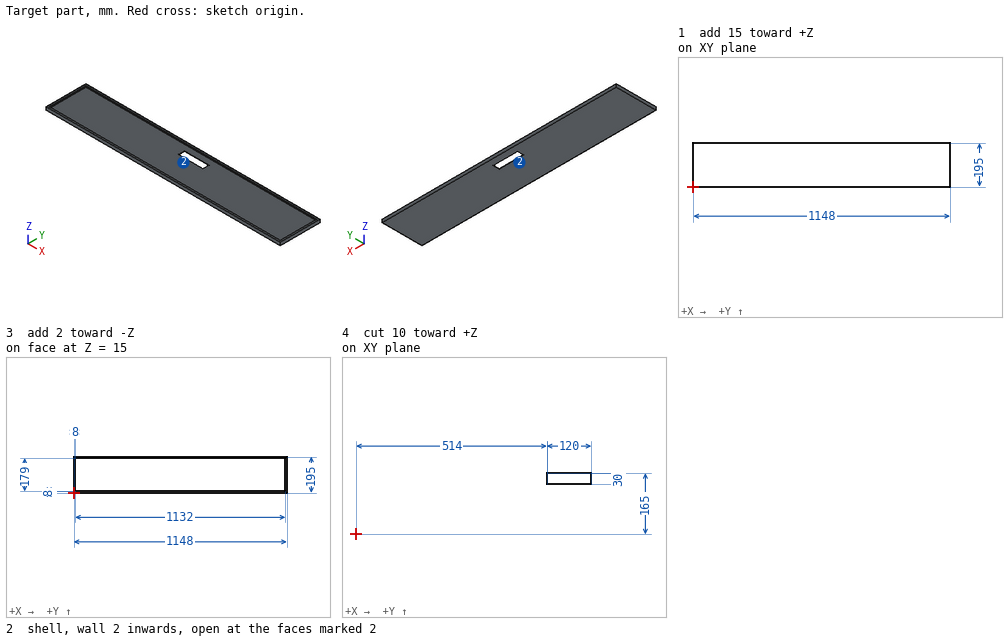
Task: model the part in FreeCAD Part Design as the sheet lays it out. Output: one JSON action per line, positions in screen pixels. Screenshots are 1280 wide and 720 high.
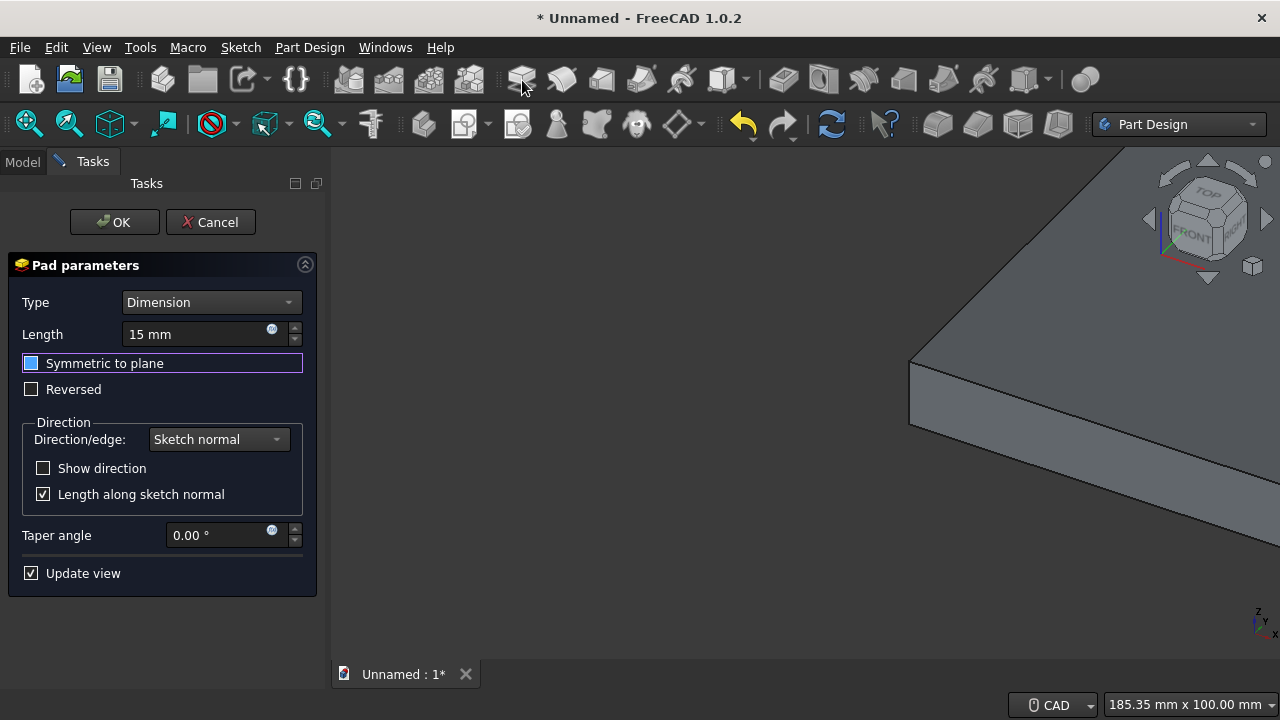
{"action": "left_click", "coordinate": [115, 222]}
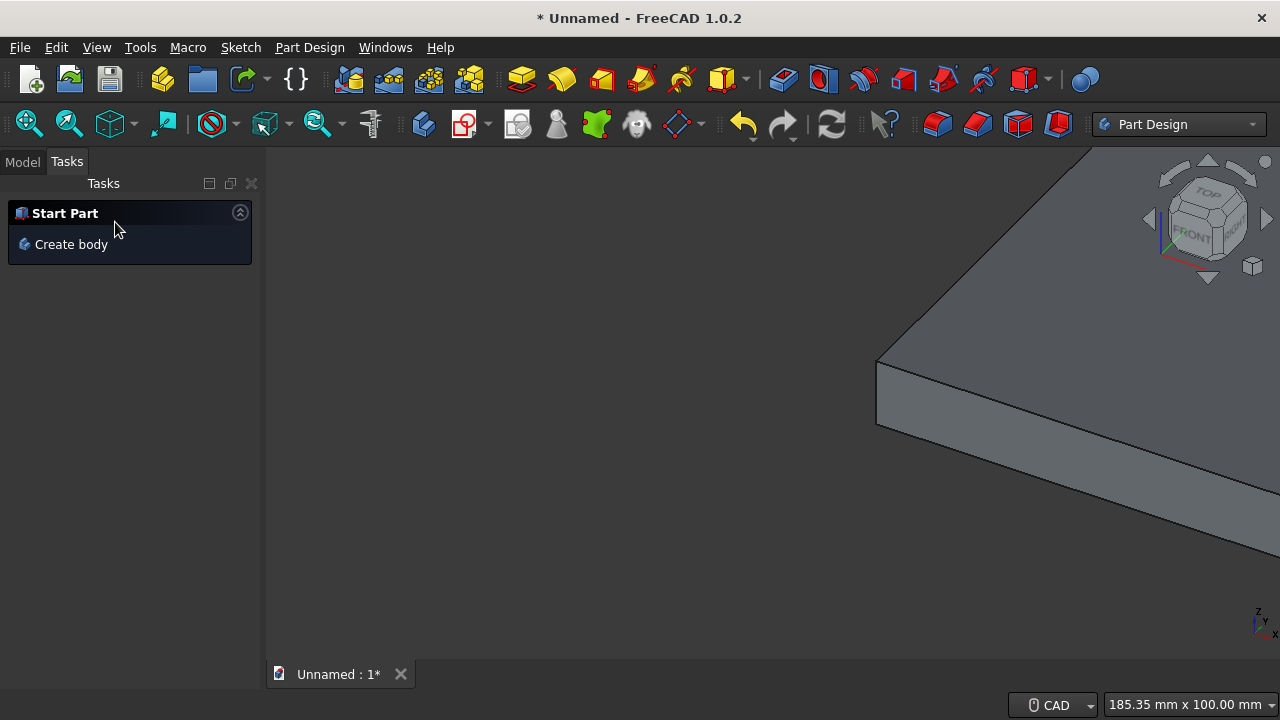
{"action": "left_click", "coordinate": [30, 124]}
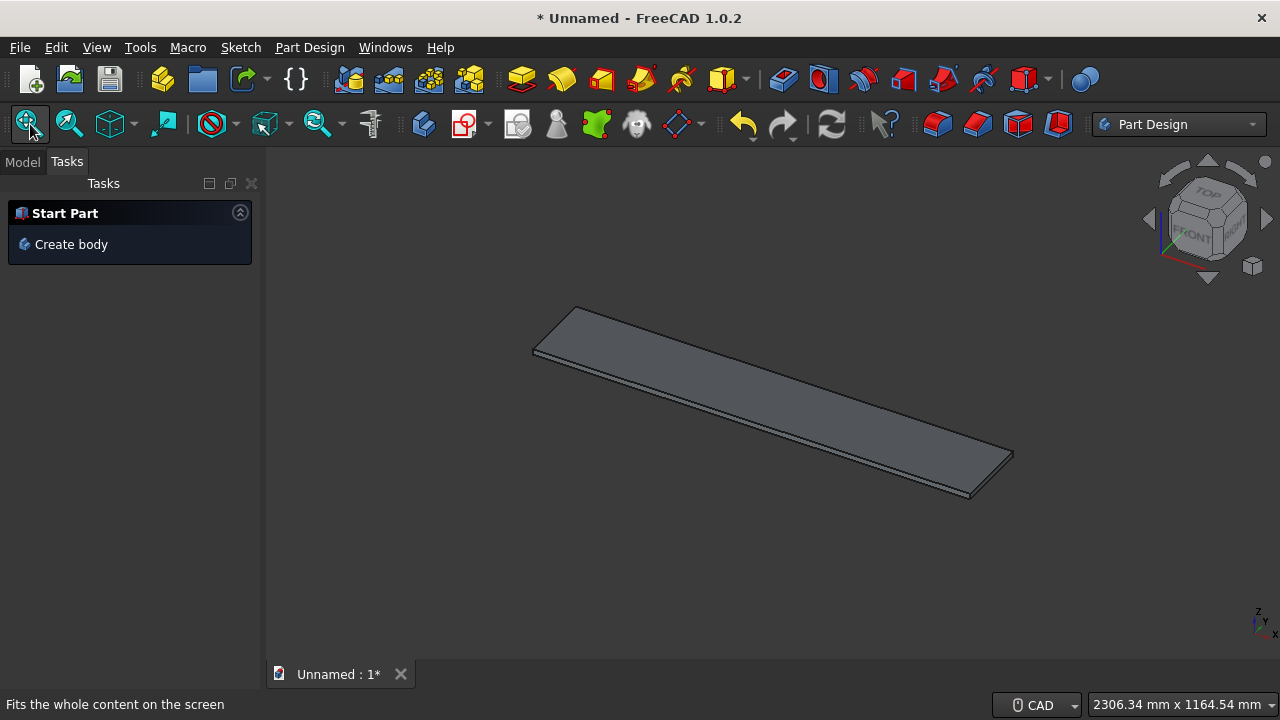
{"action": "left_click", "coordinate": [898, 441]}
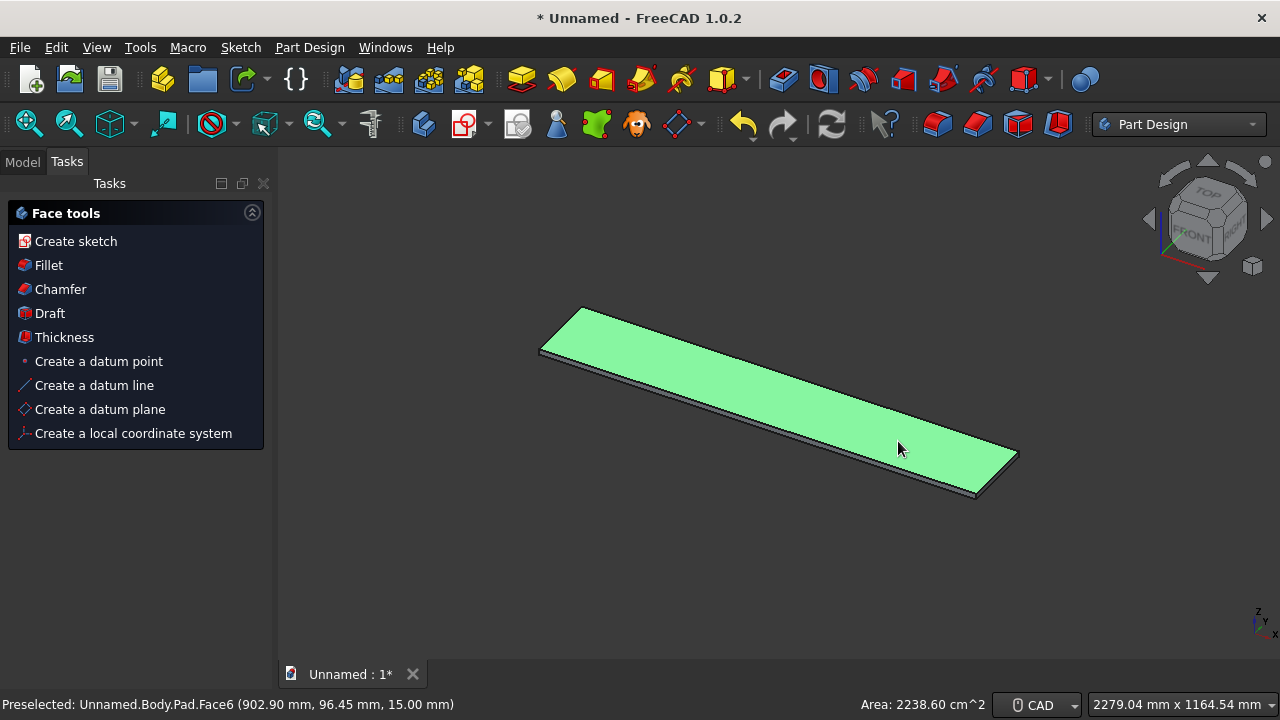
{"action": "left_click", "coordinate": [1058, 124]}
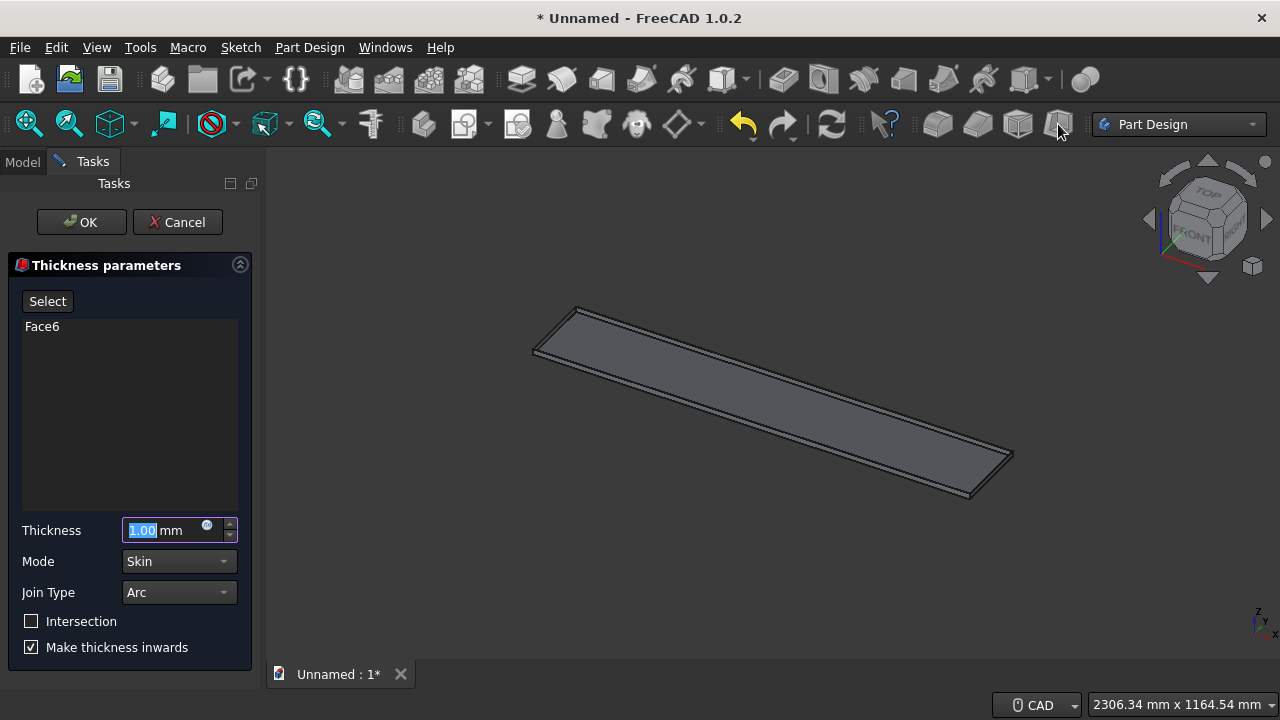
{"action": "type", "text": "2"}
{"action": "key", "text": "Tab"}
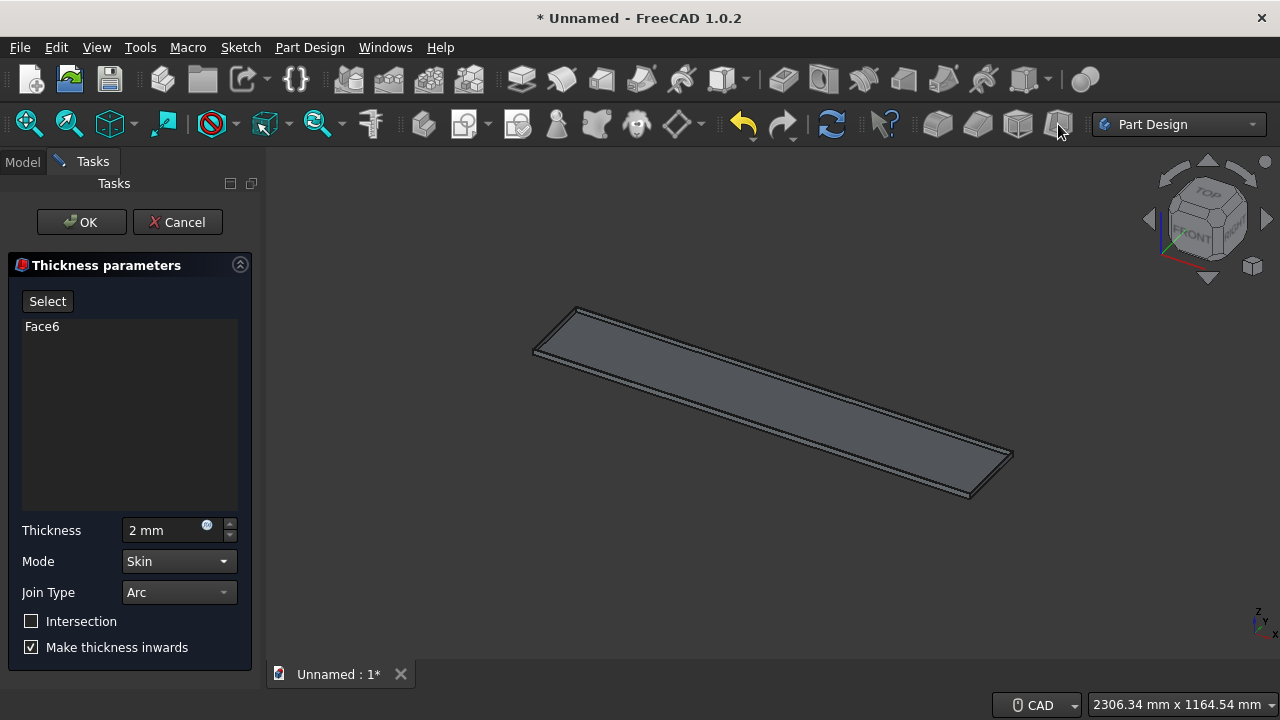
{"action": "left_click", "coordinate": [180, 592]}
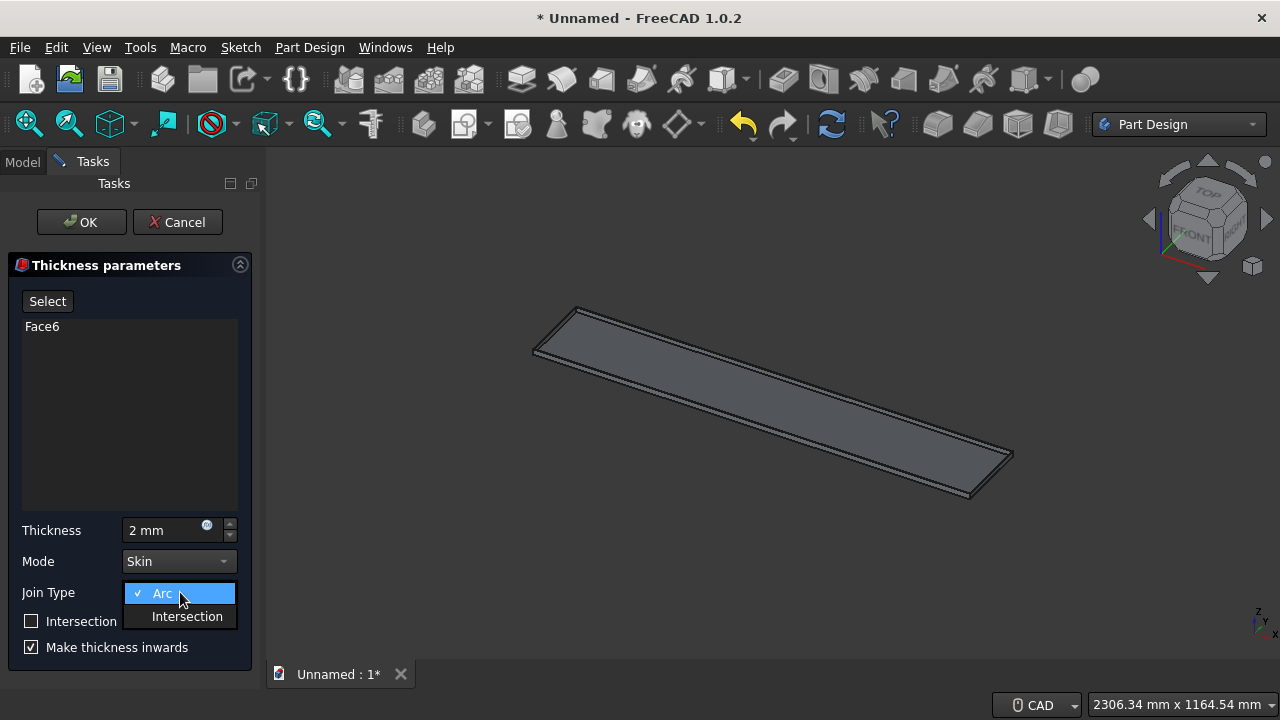
{"action": "left_click", "coordinate": [179, 616]}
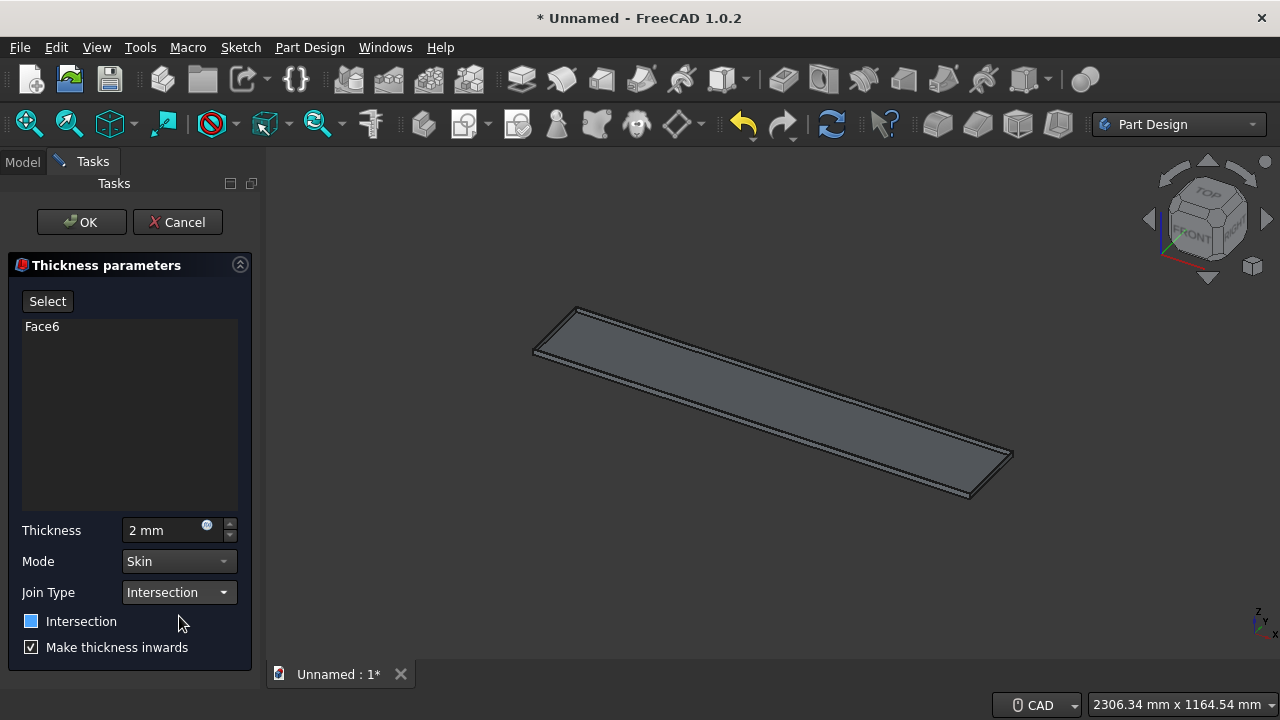
{"action": "left_click", "coordinate": [82, 222]}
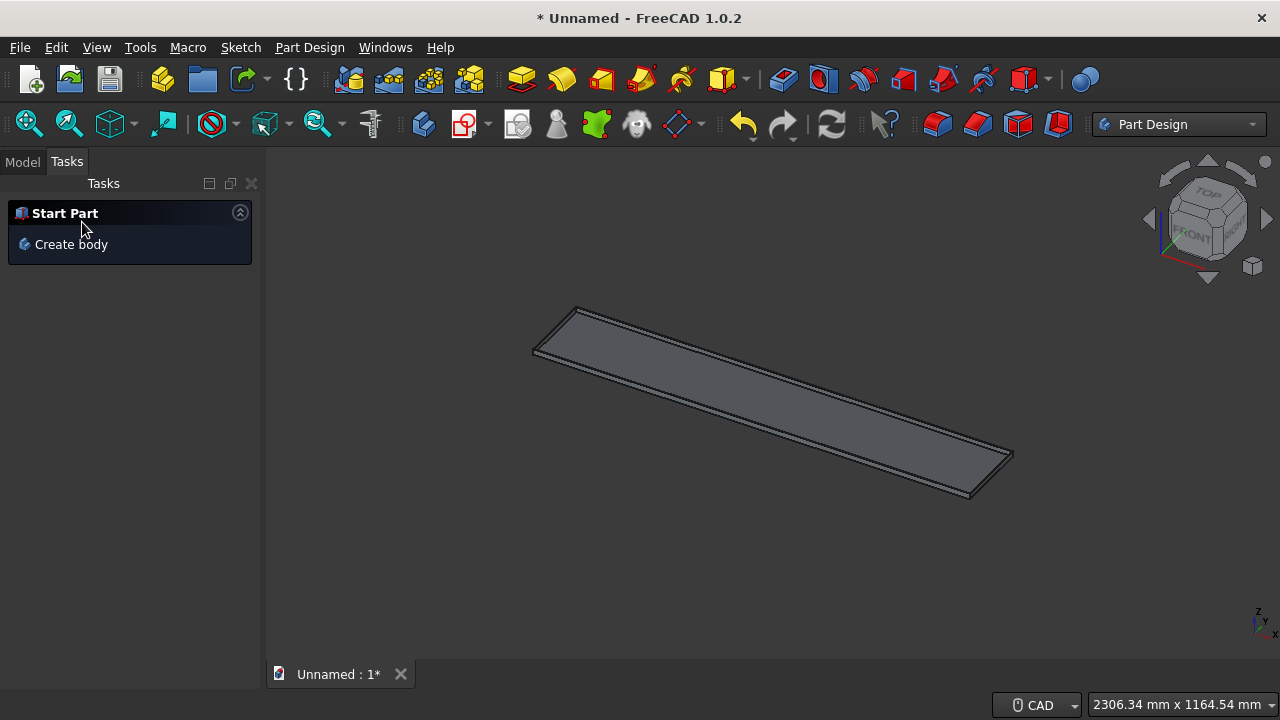
{"action": "scroll", "coordinate": [998, 465], "scroll_direction": "up", "scroll_amount": 15}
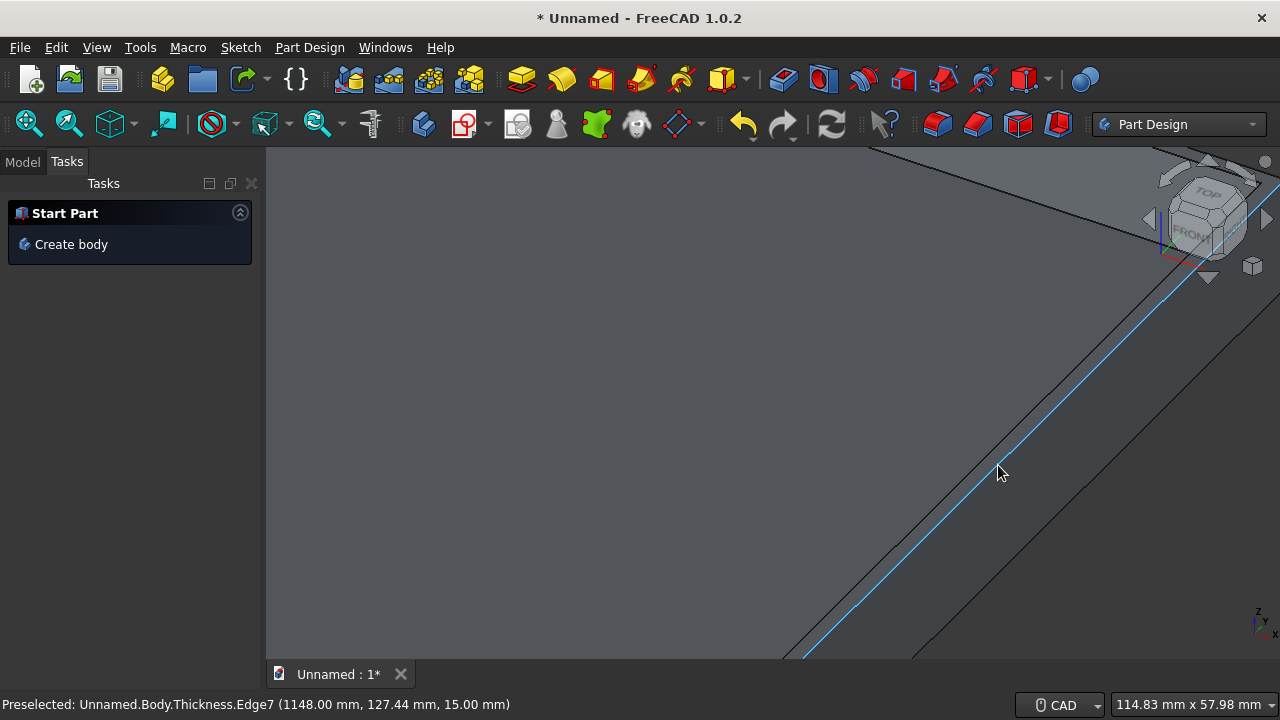
{"action": "scroll", "coordinate": [990, 465], "scroll_direction": "up", "scroll_amount": 4}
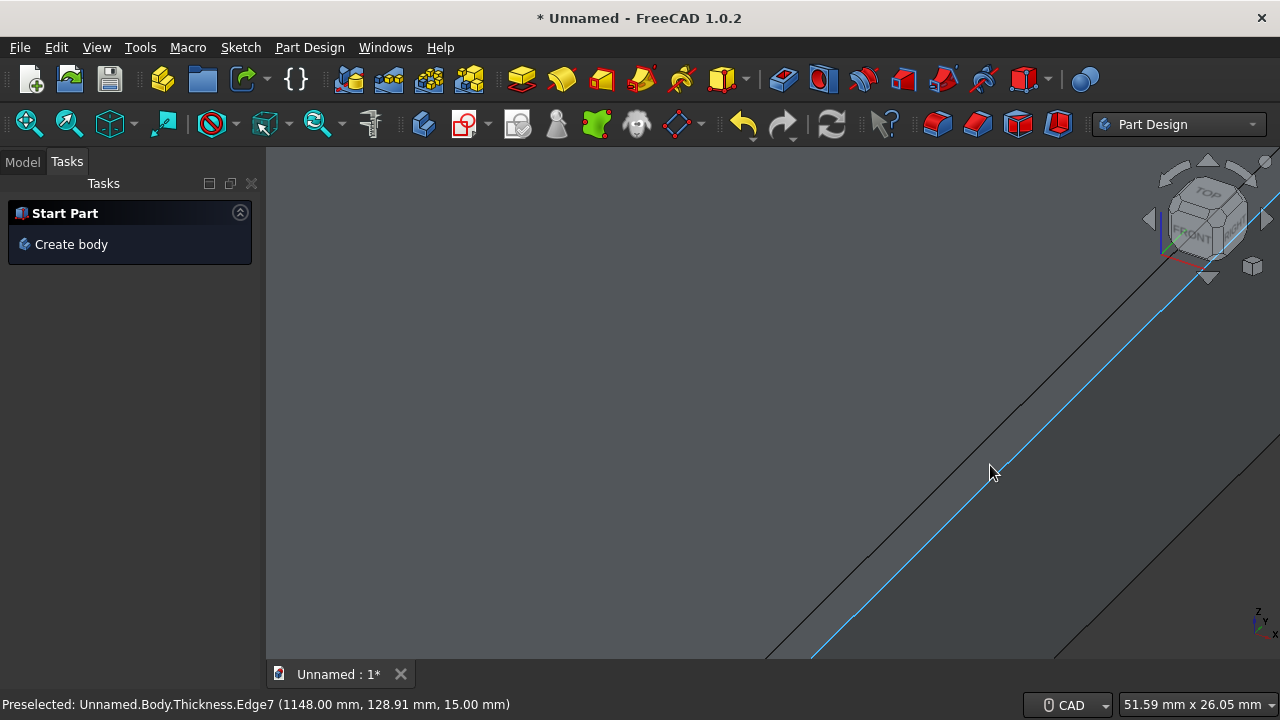
{"action": "left_click", "coordinate": [990, 465]}